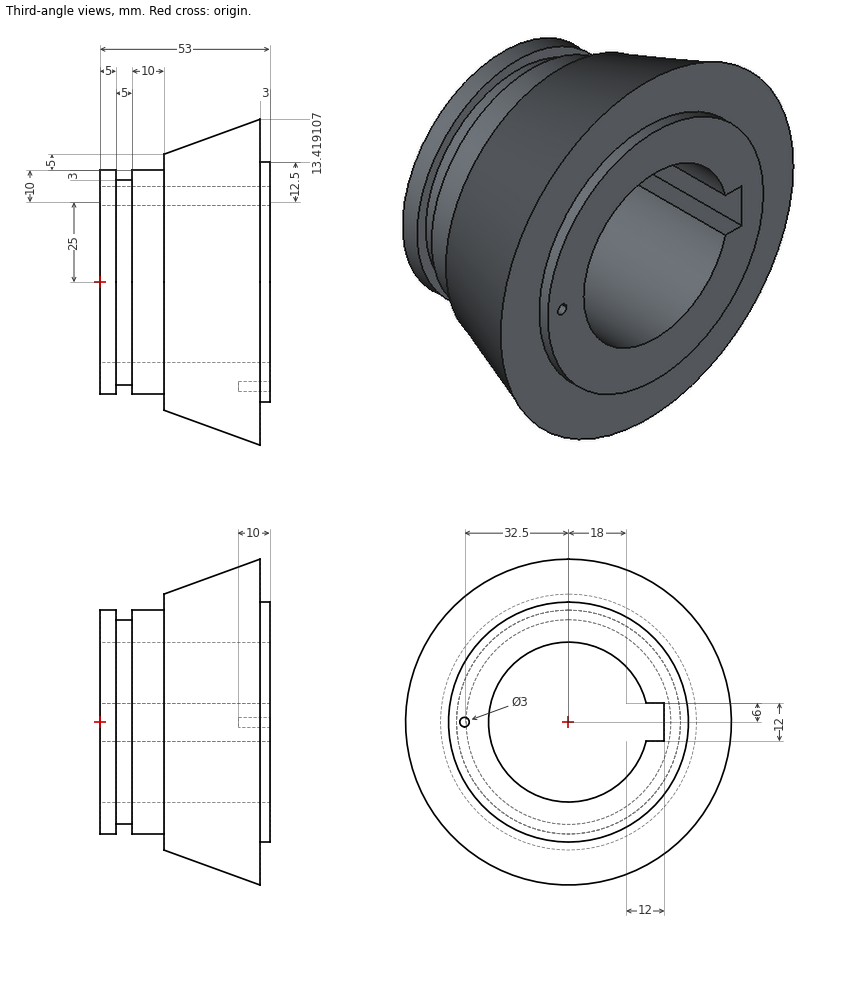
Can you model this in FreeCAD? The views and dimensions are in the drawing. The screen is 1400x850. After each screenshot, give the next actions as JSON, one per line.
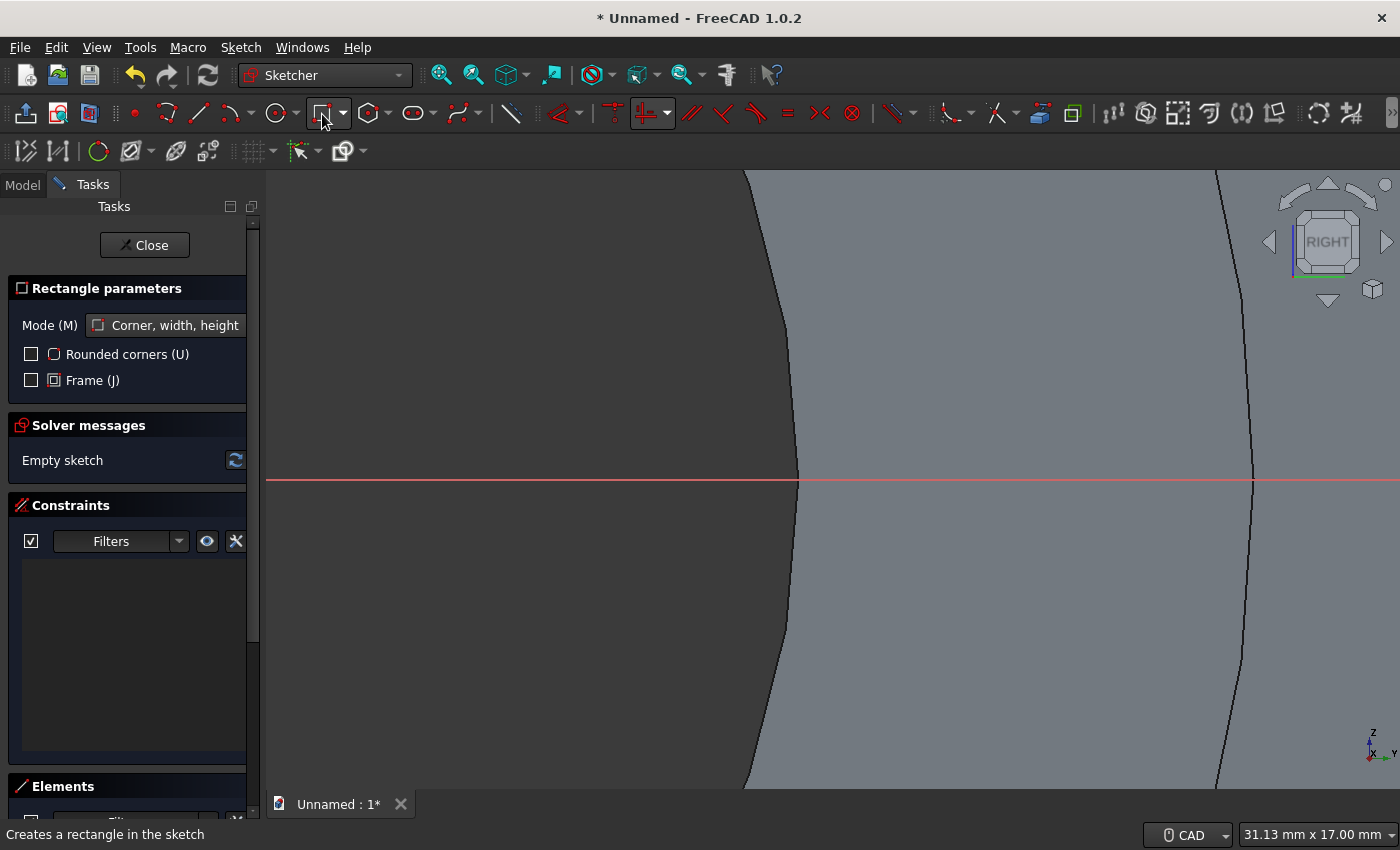
{"action": "left_click", "coordinate": [543, 261]}
{"action": "mouse_move", "coordinate": [980, 698]}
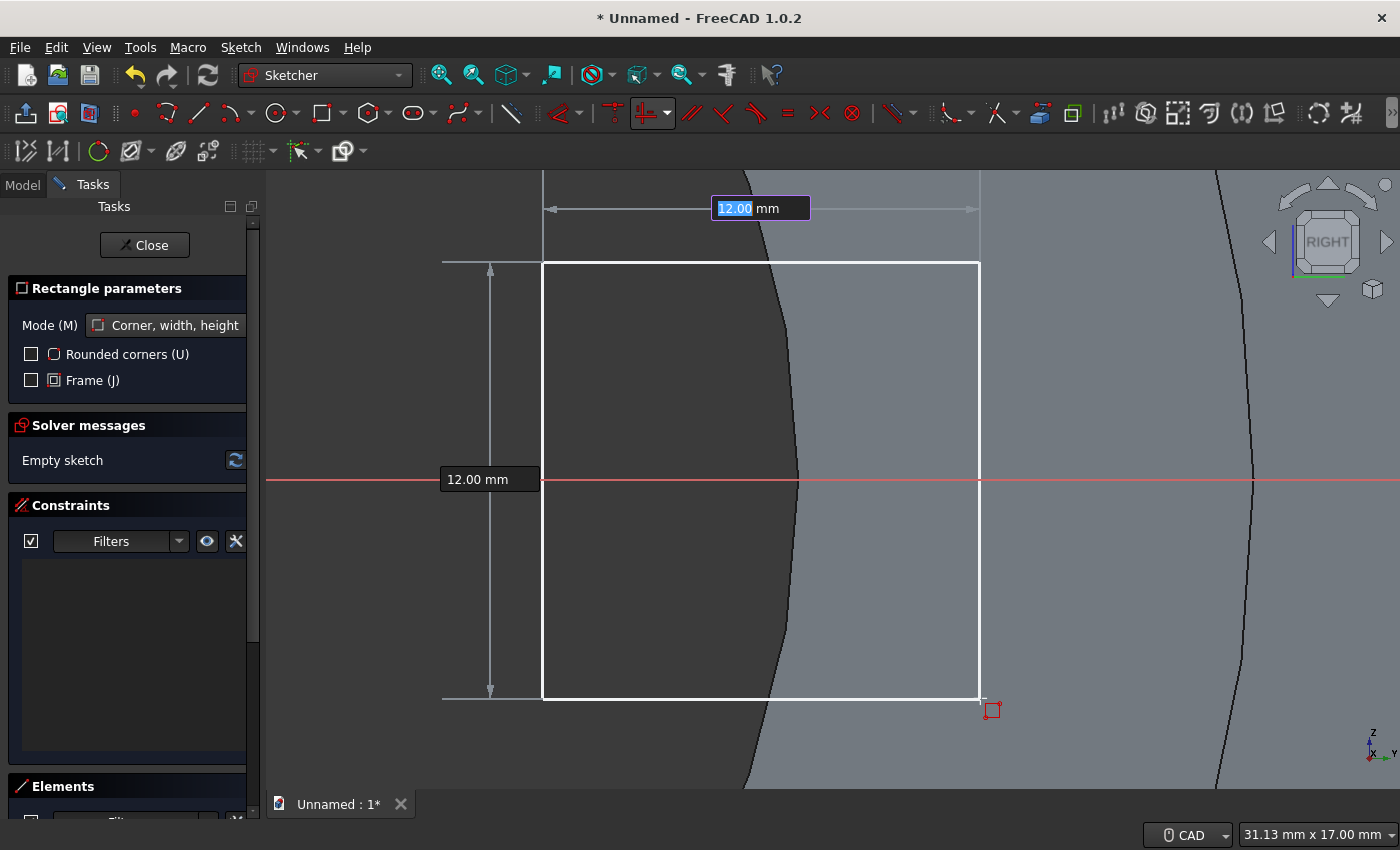
{"action": "type", "text": "12"}
{"action": "key", "text": "Tab"}
{"action": "type", "text": "12"}
{"action": "key", "text": "Return"}
{"action": "key", "text": "Escape"}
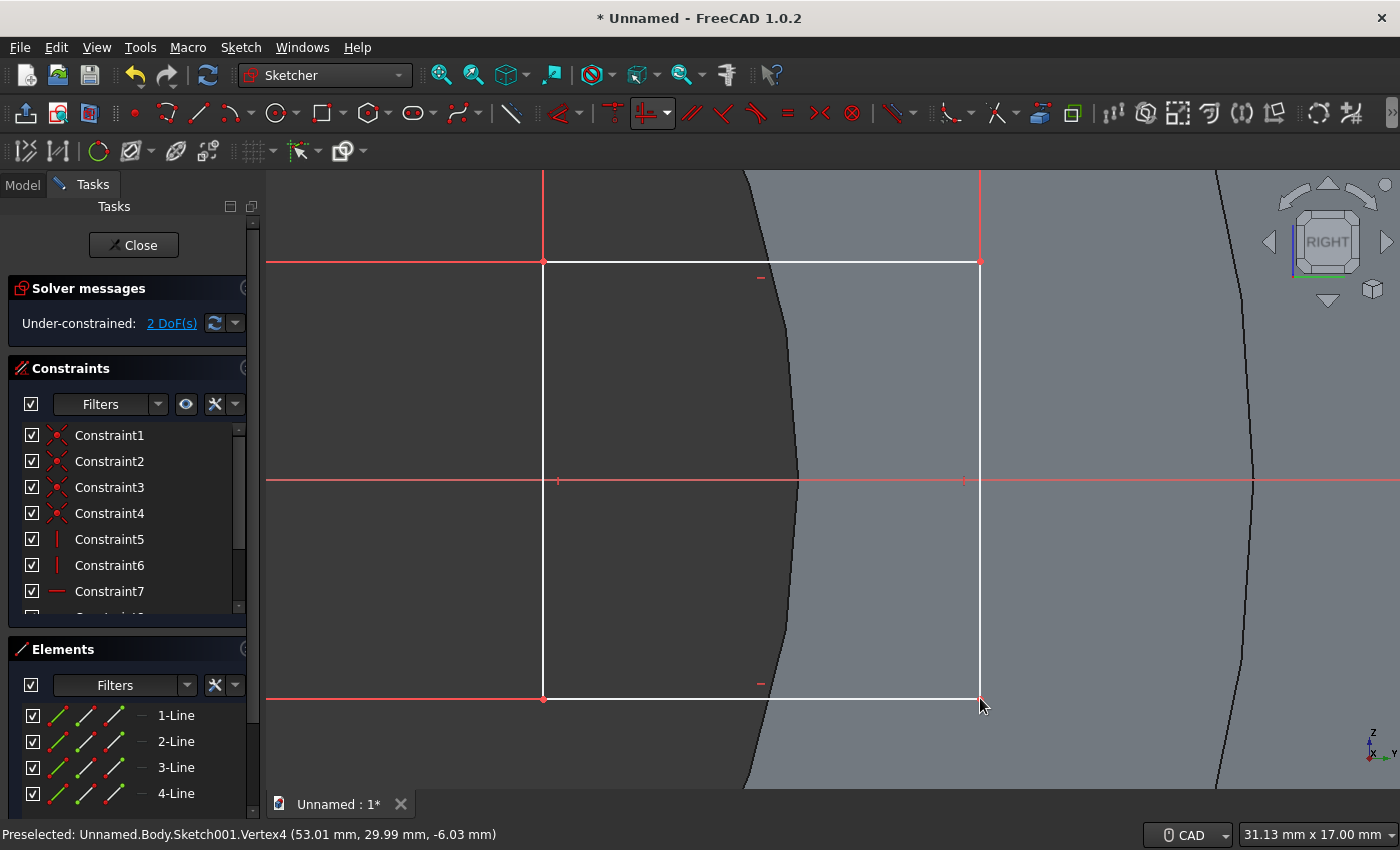
{"action": "left_click", "coordinate": [558, 114]}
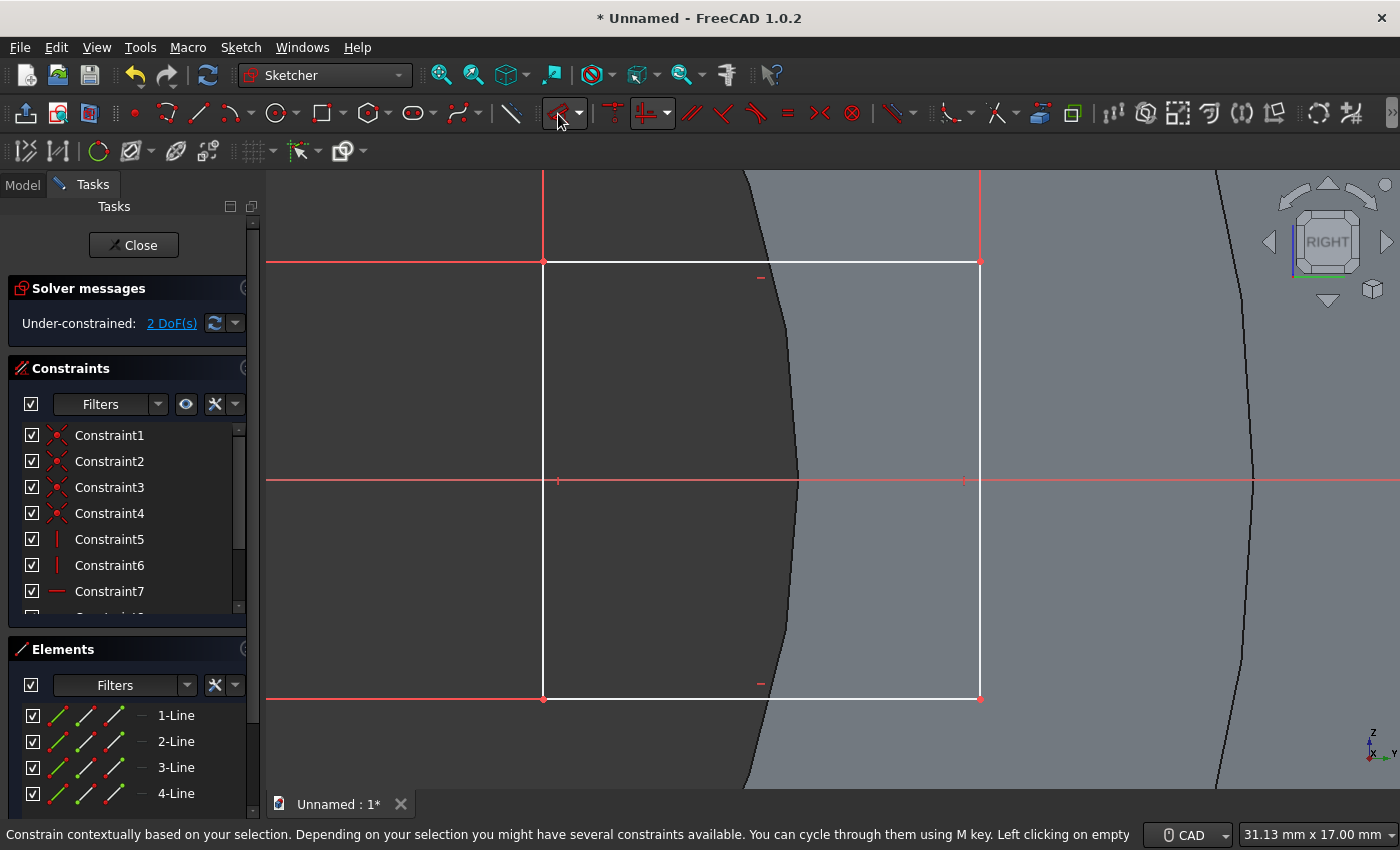
{"action": "left_click", "coordinate": [543, 262]}
{"action": "left_click", "coordinate": [577, 371]}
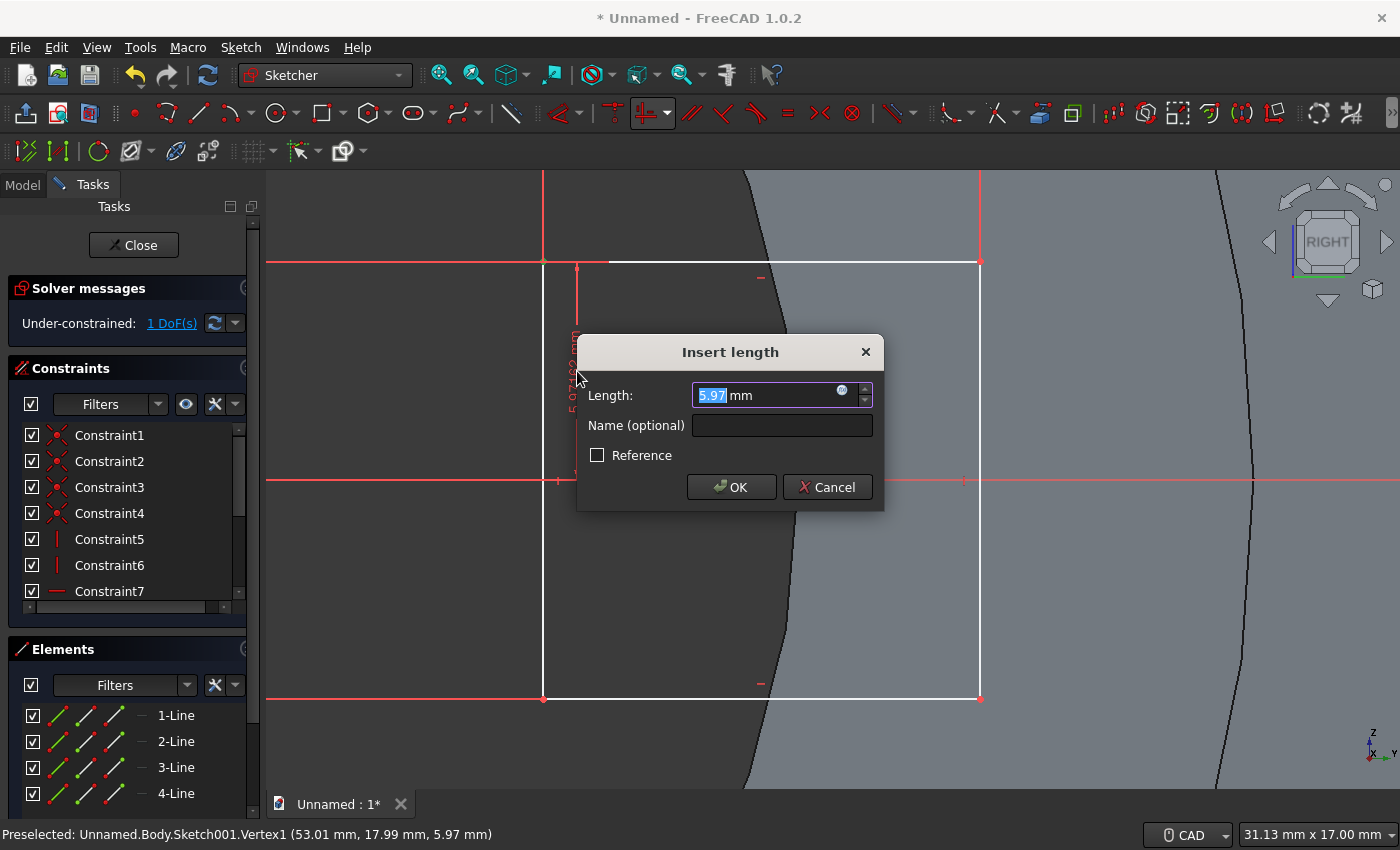
{"action": "type", "text": "6"}
{"action": "key", "text": "Return"}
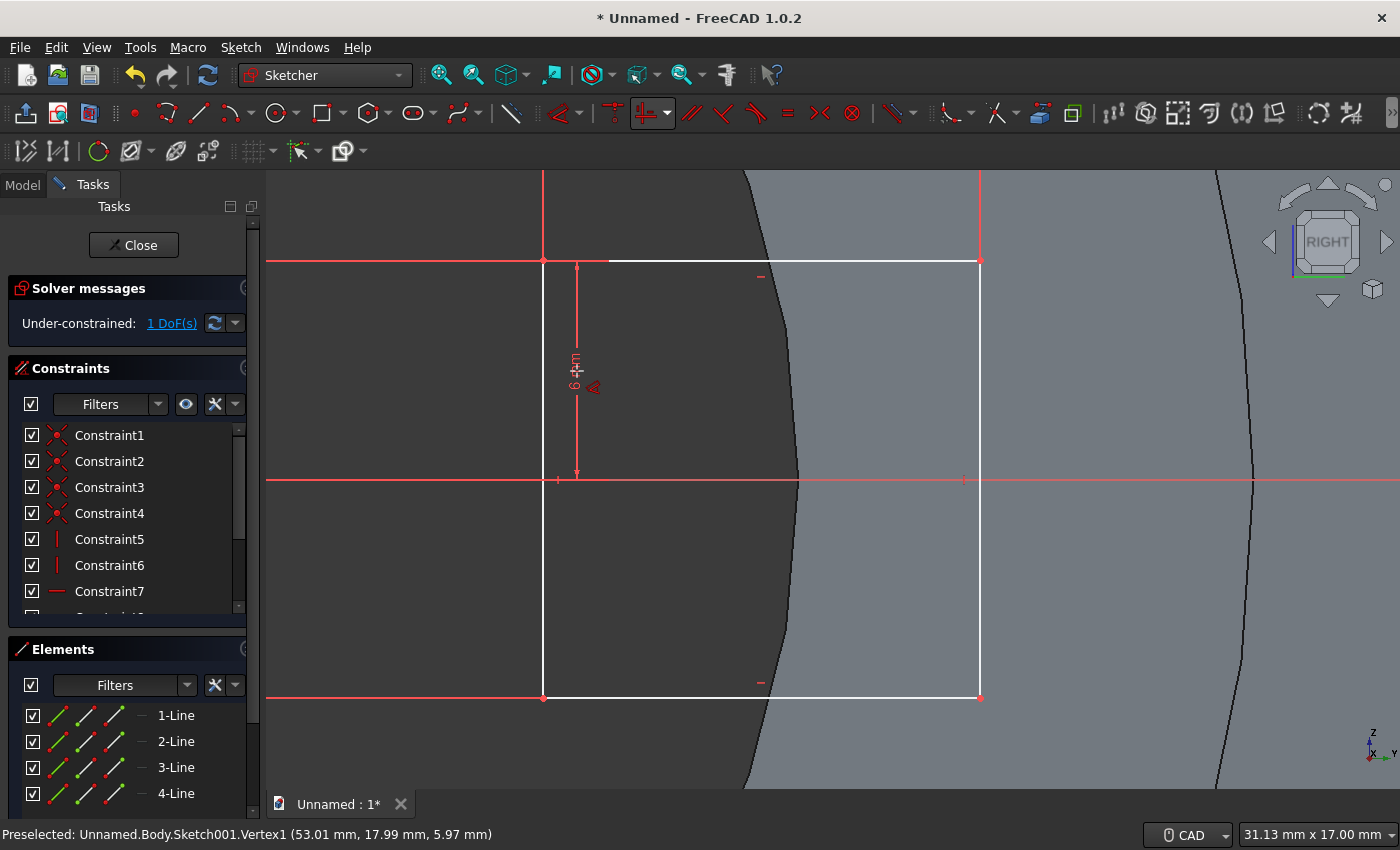
{"action": "left_click", "coordinate": [543, 261]}
{"action": "left_click", "coordinate": [418, 227]}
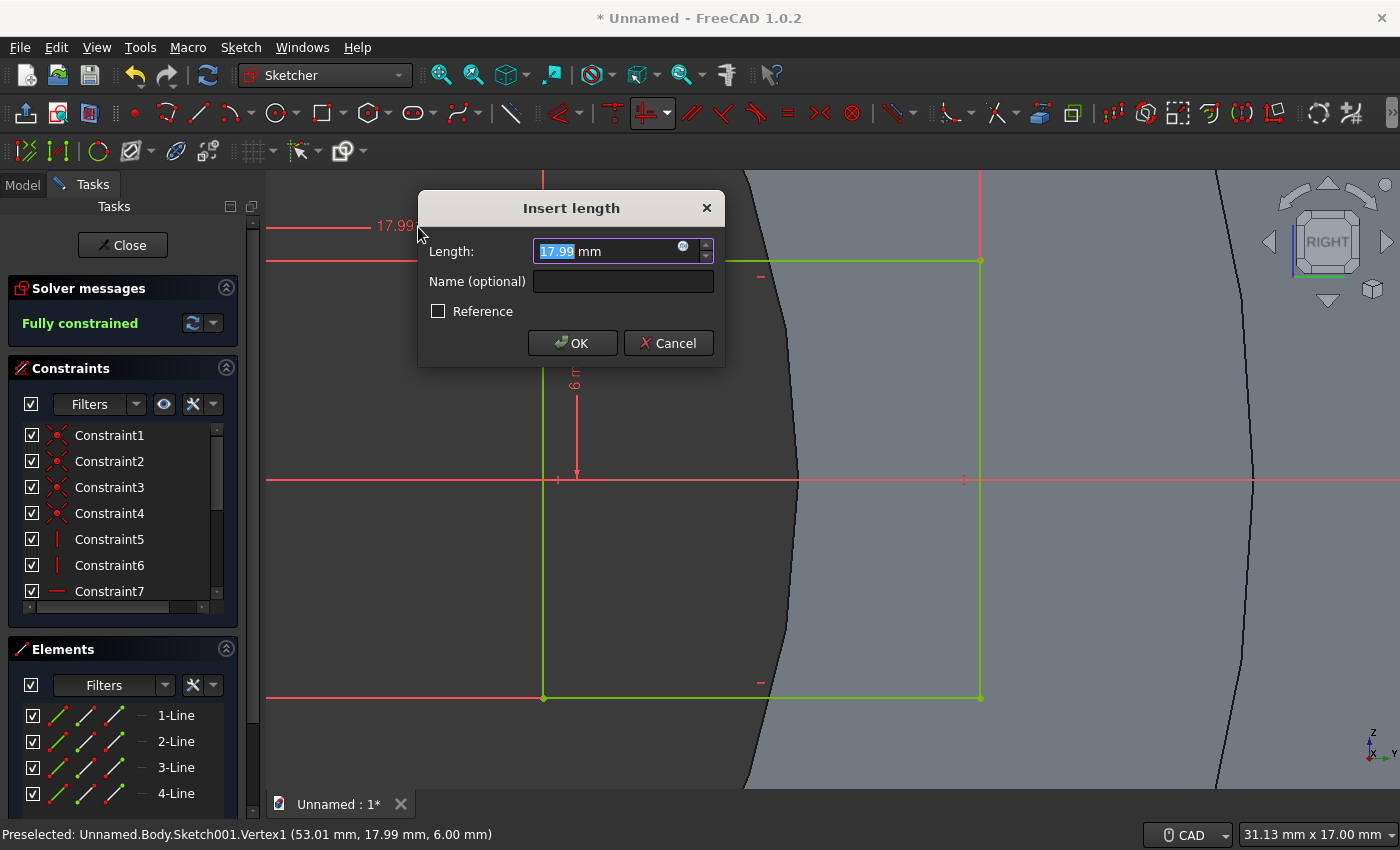
{"action": "type", "text": "18"}
{"action": "key", "text": "Return"}
{"action": "key", "text": "Escape"}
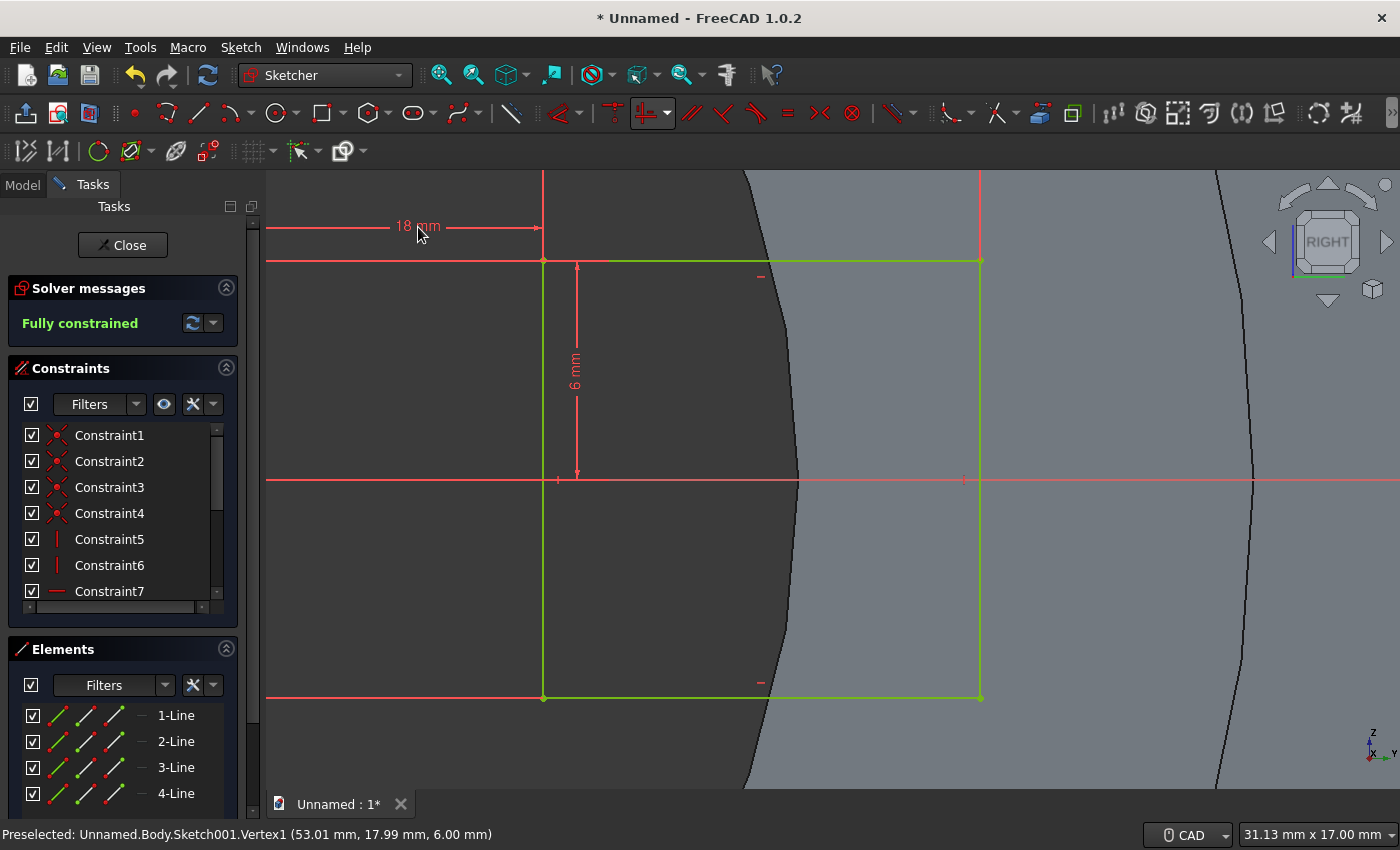
{"action": "left_click", "coordinate": [123, 245]}